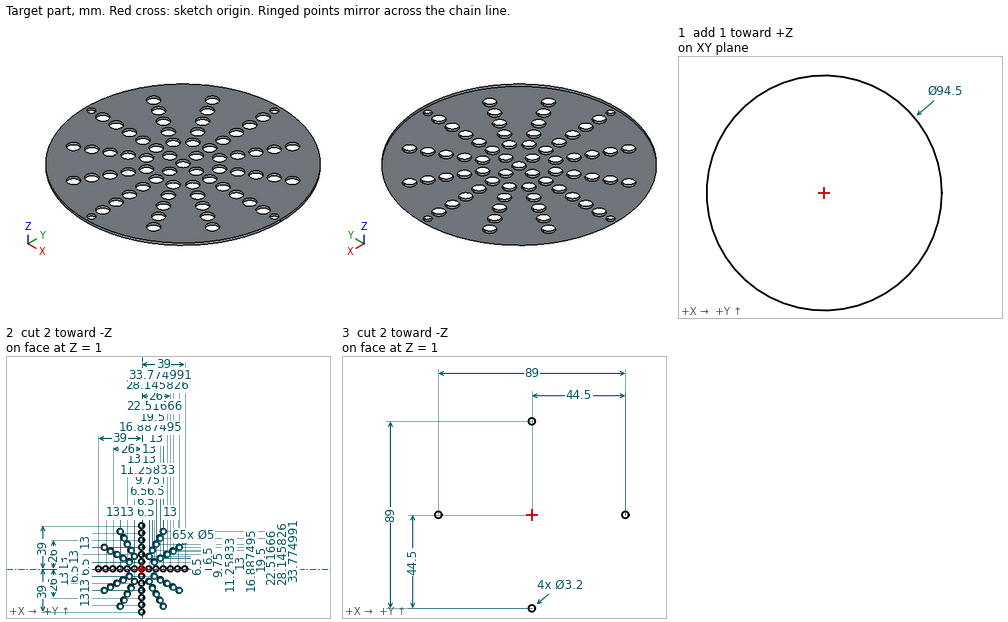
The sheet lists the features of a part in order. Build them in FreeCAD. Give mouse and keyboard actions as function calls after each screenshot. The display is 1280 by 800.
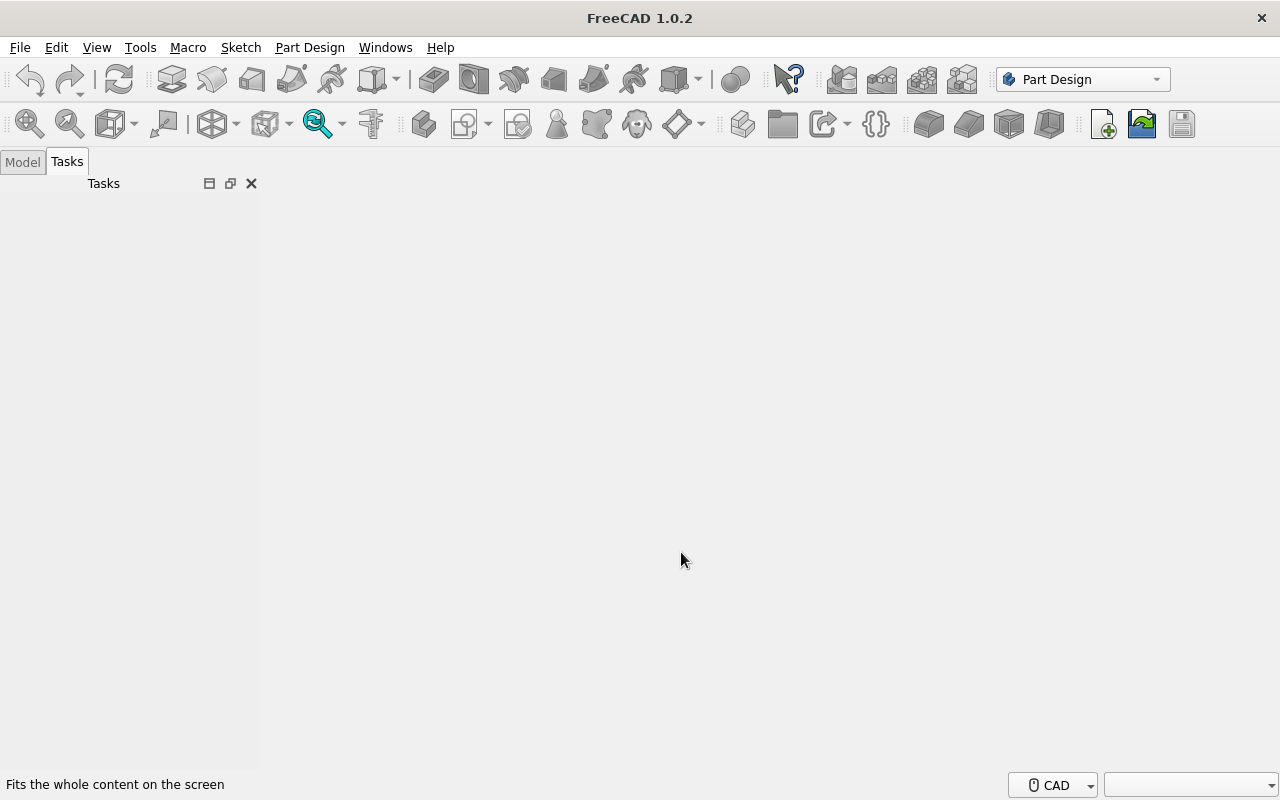
click(1102, 124)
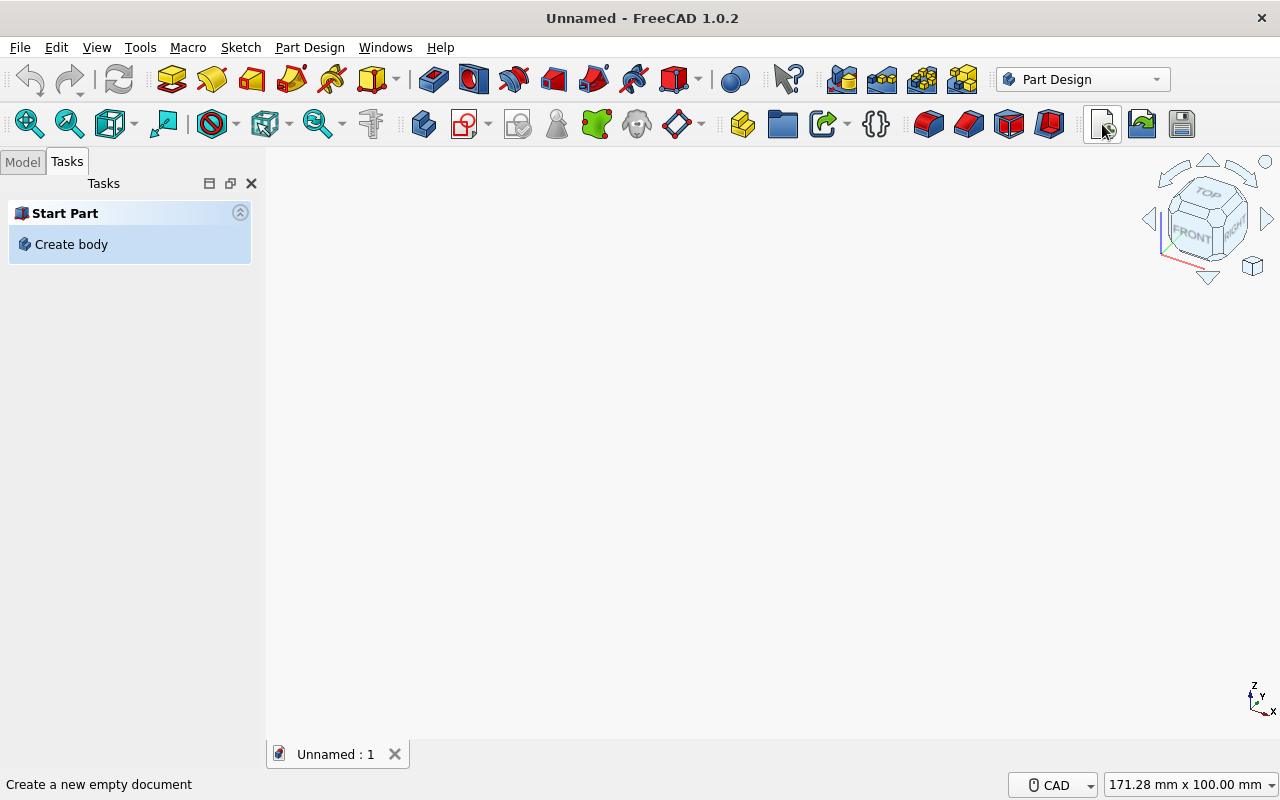
click(464, 124)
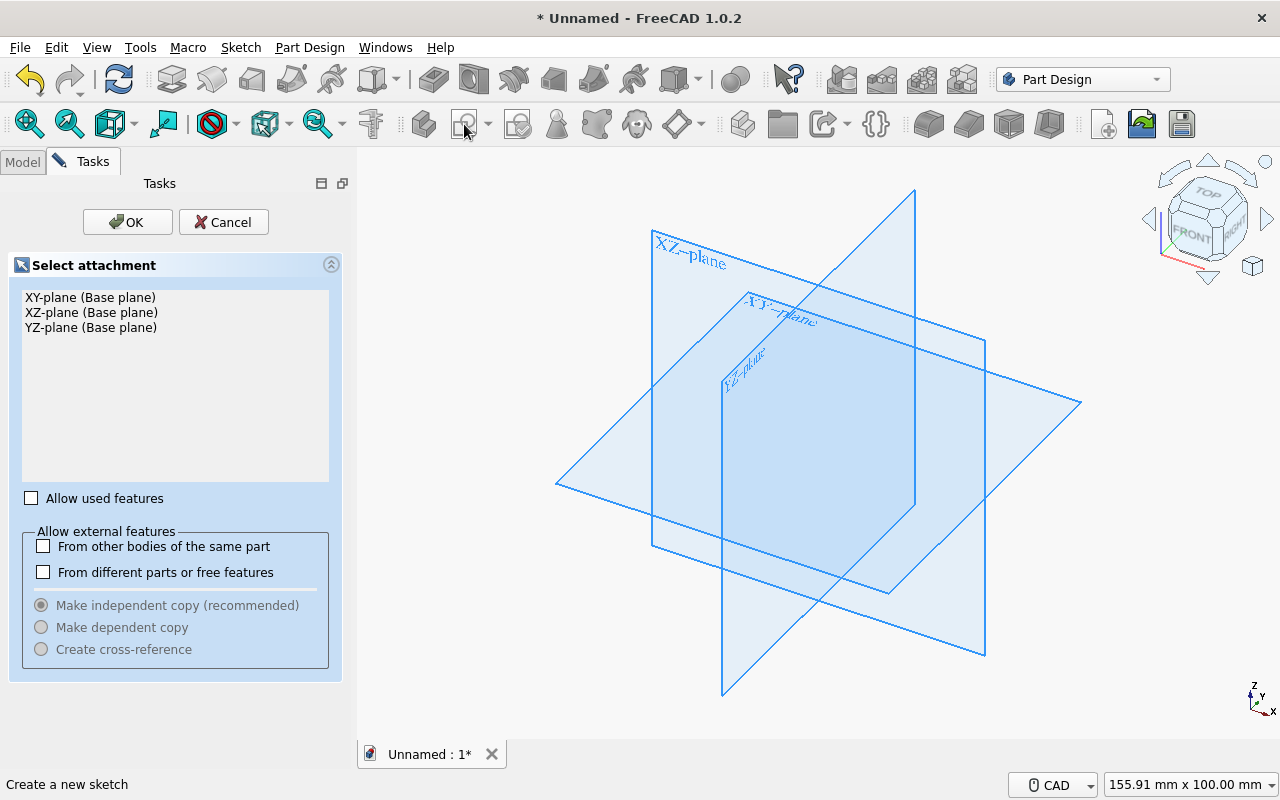
click(82, 298)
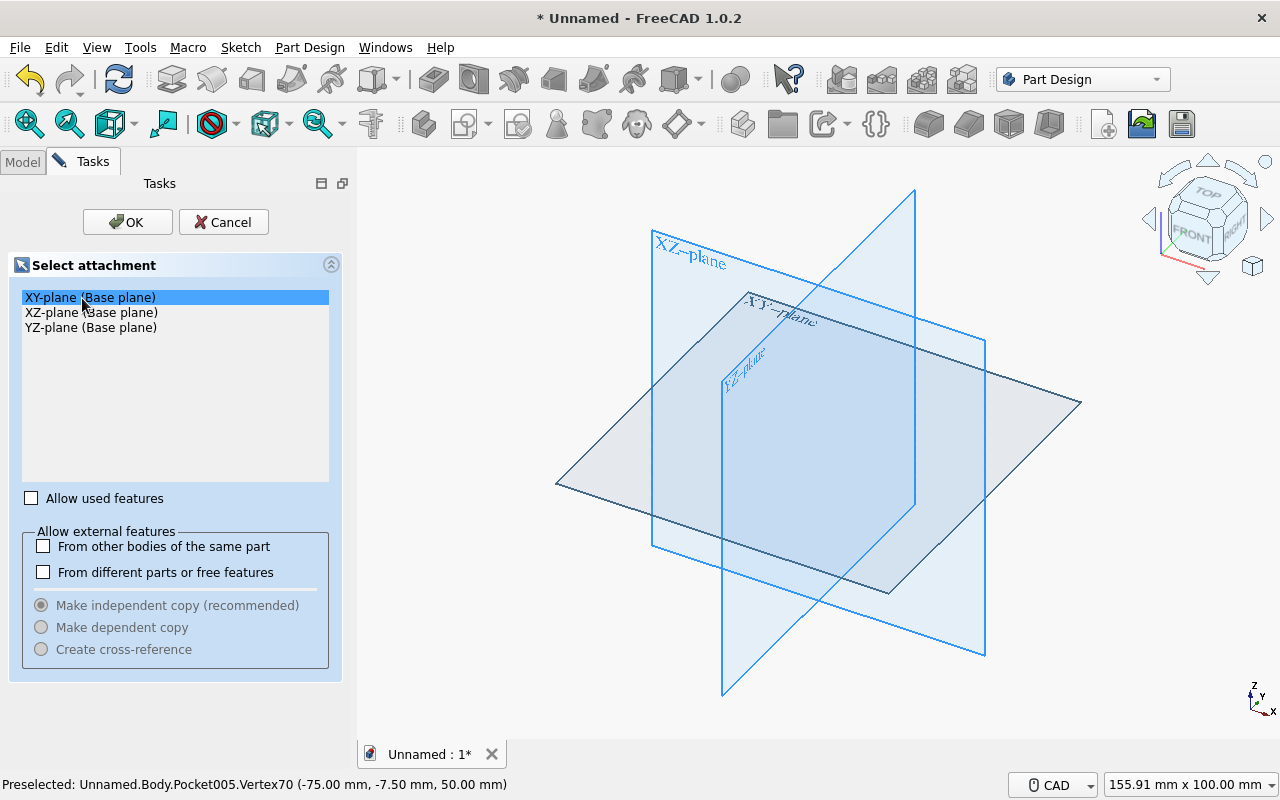
click(128, 222)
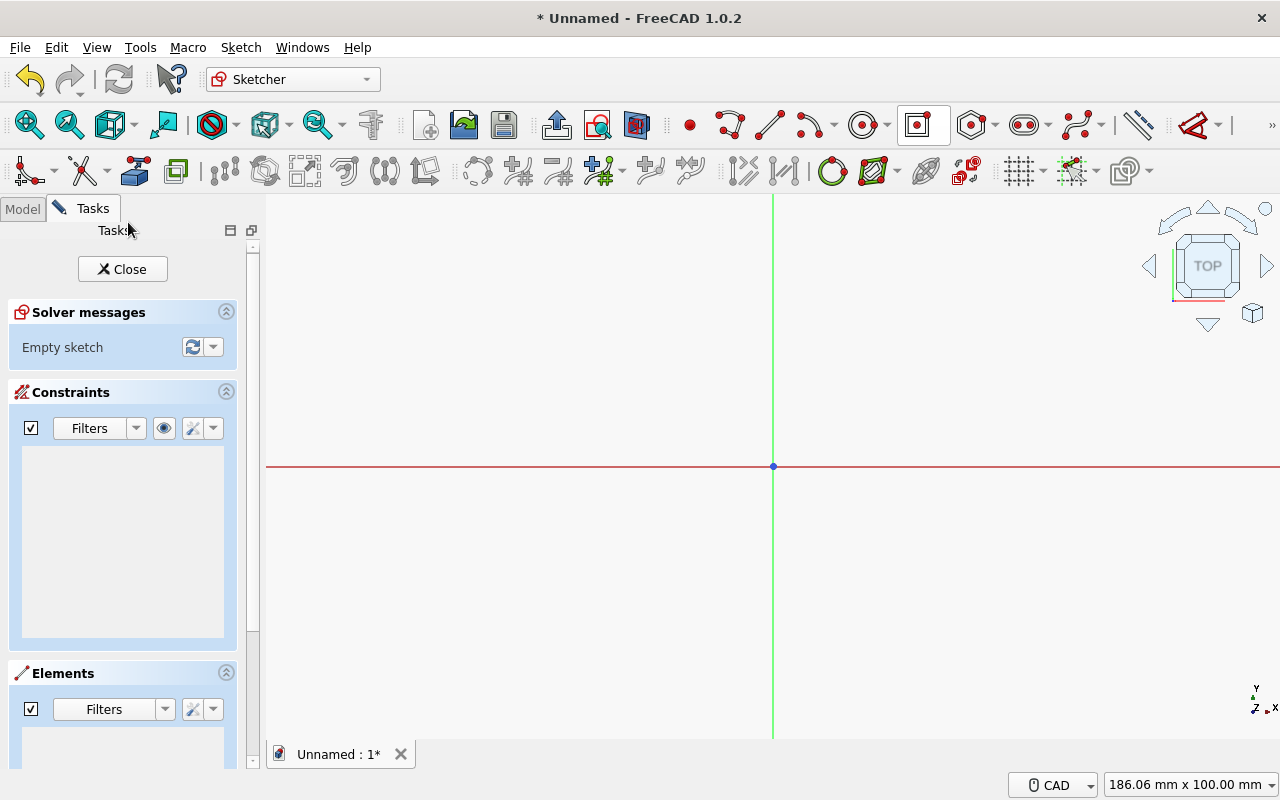
scroll(565, 466, down, 2)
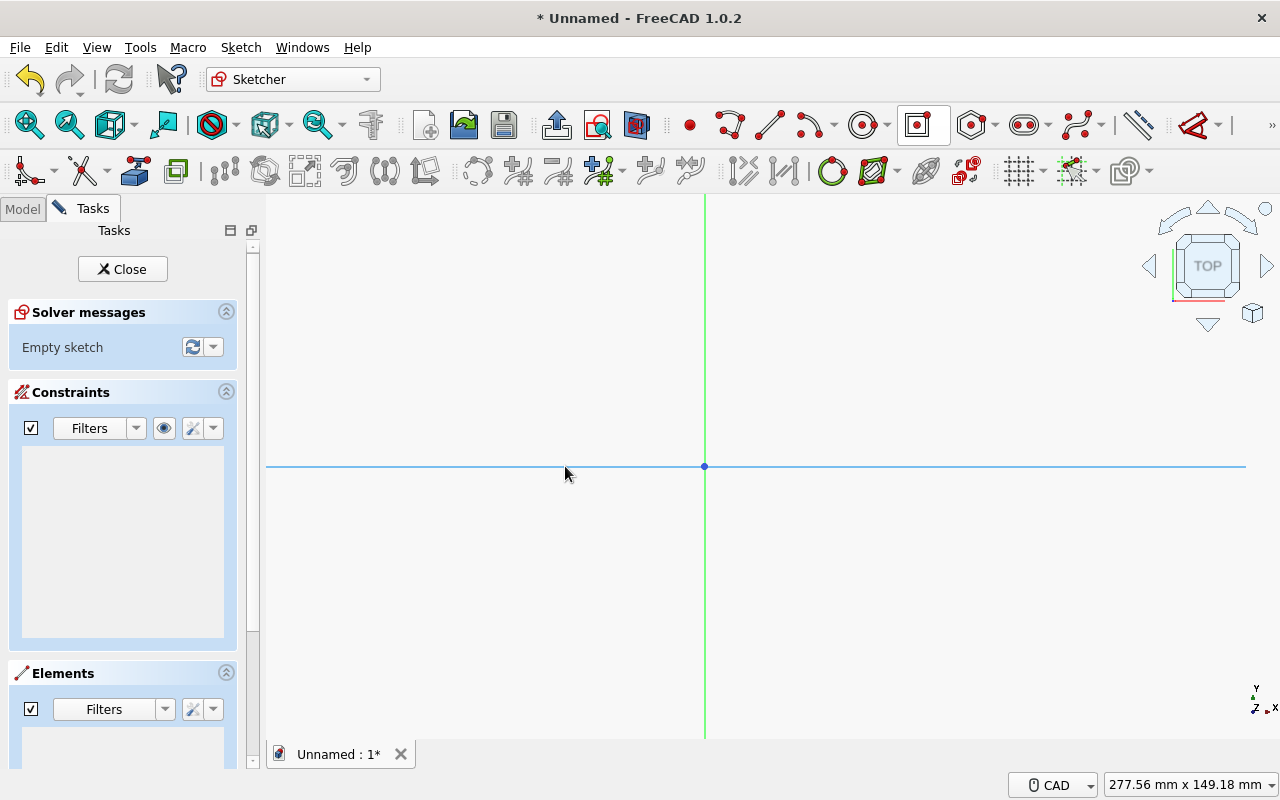
key(g)
key(c)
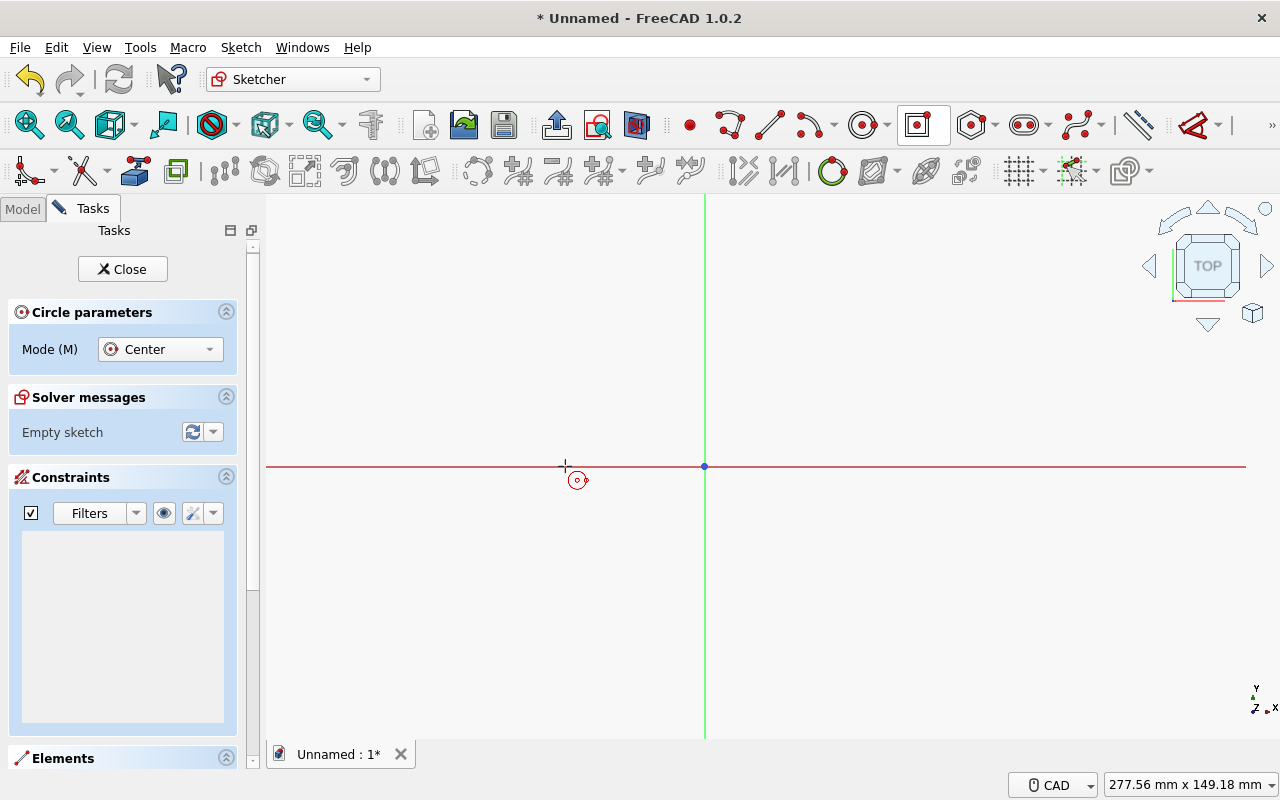
click(705, 466)
move(827, 344)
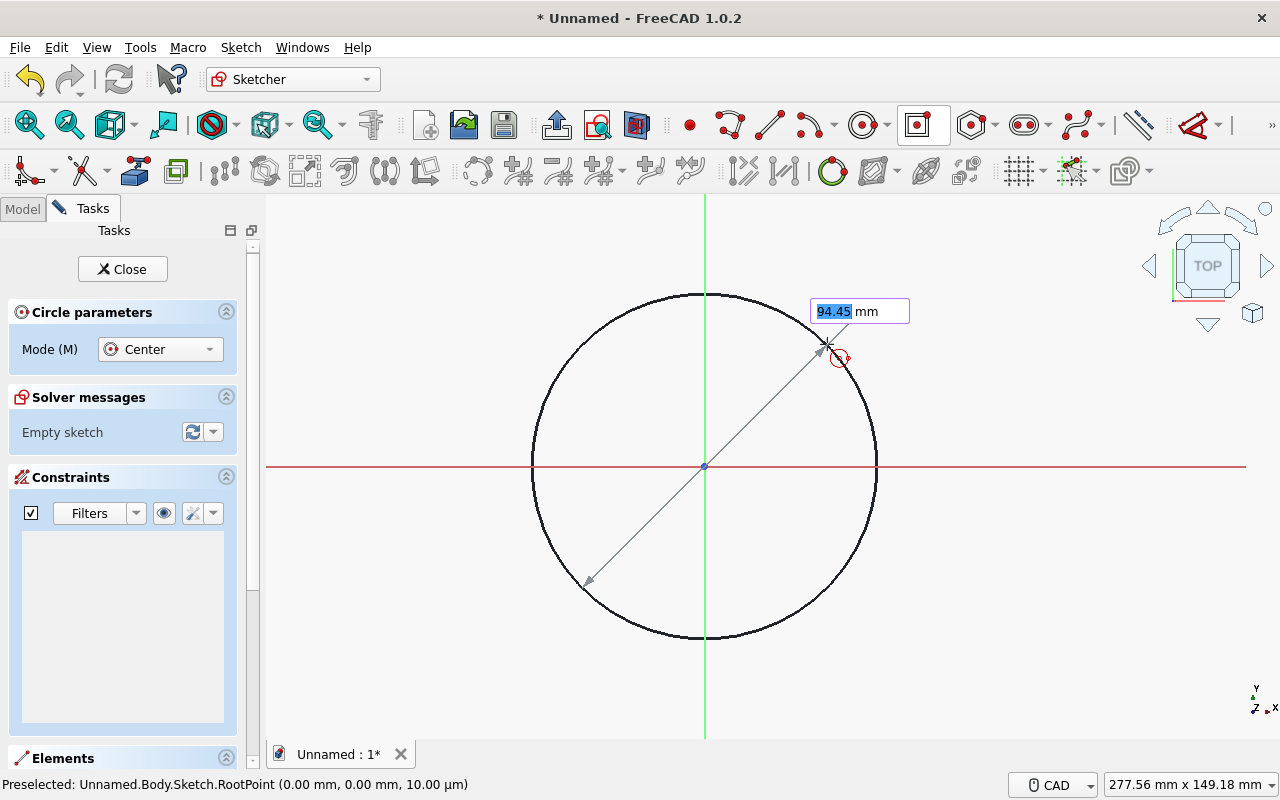
text(94.5)
key(Return)
key(Escape)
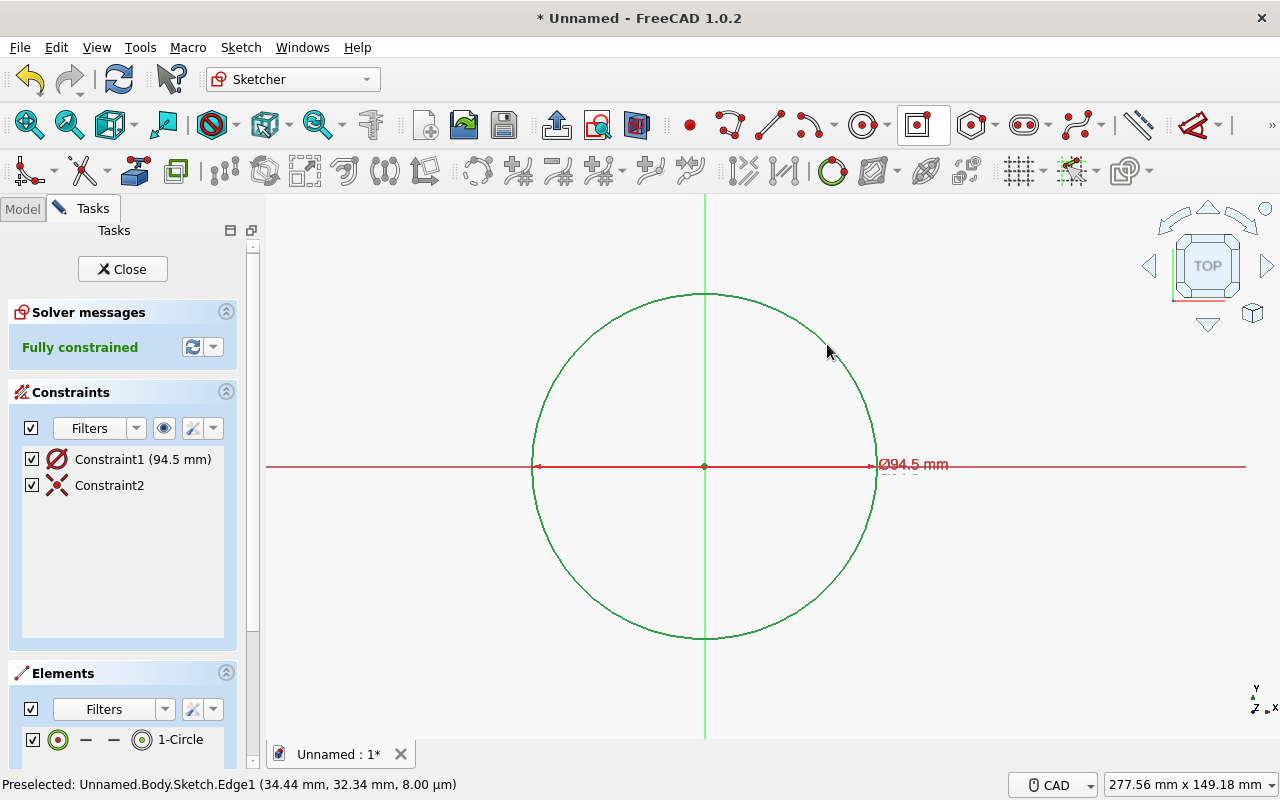
click(123, 269)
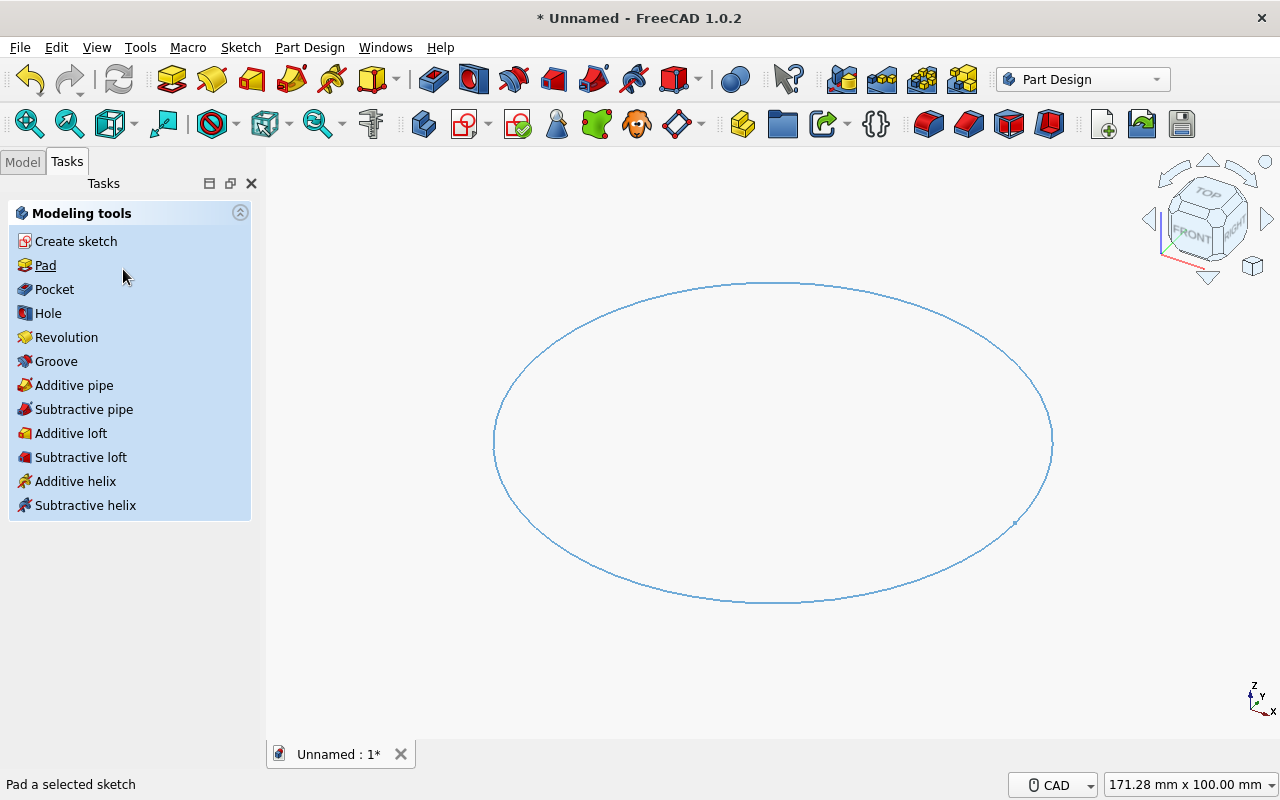
click(172, 80)